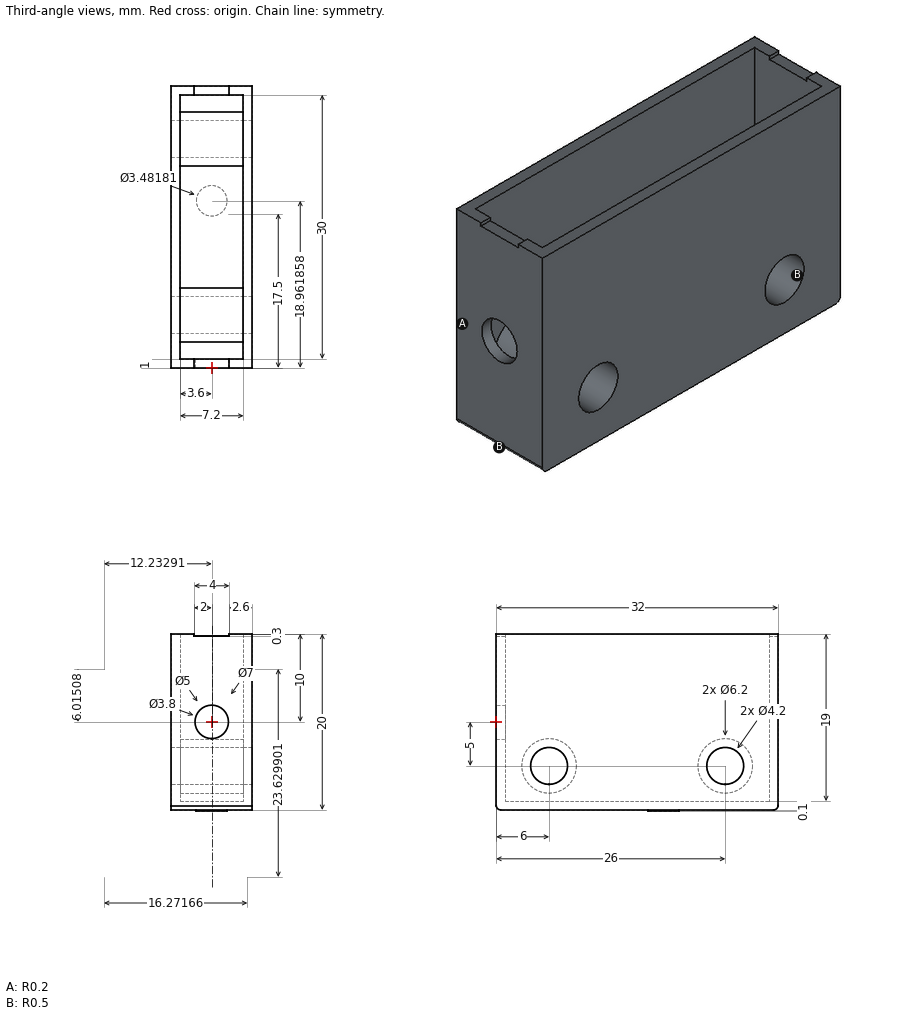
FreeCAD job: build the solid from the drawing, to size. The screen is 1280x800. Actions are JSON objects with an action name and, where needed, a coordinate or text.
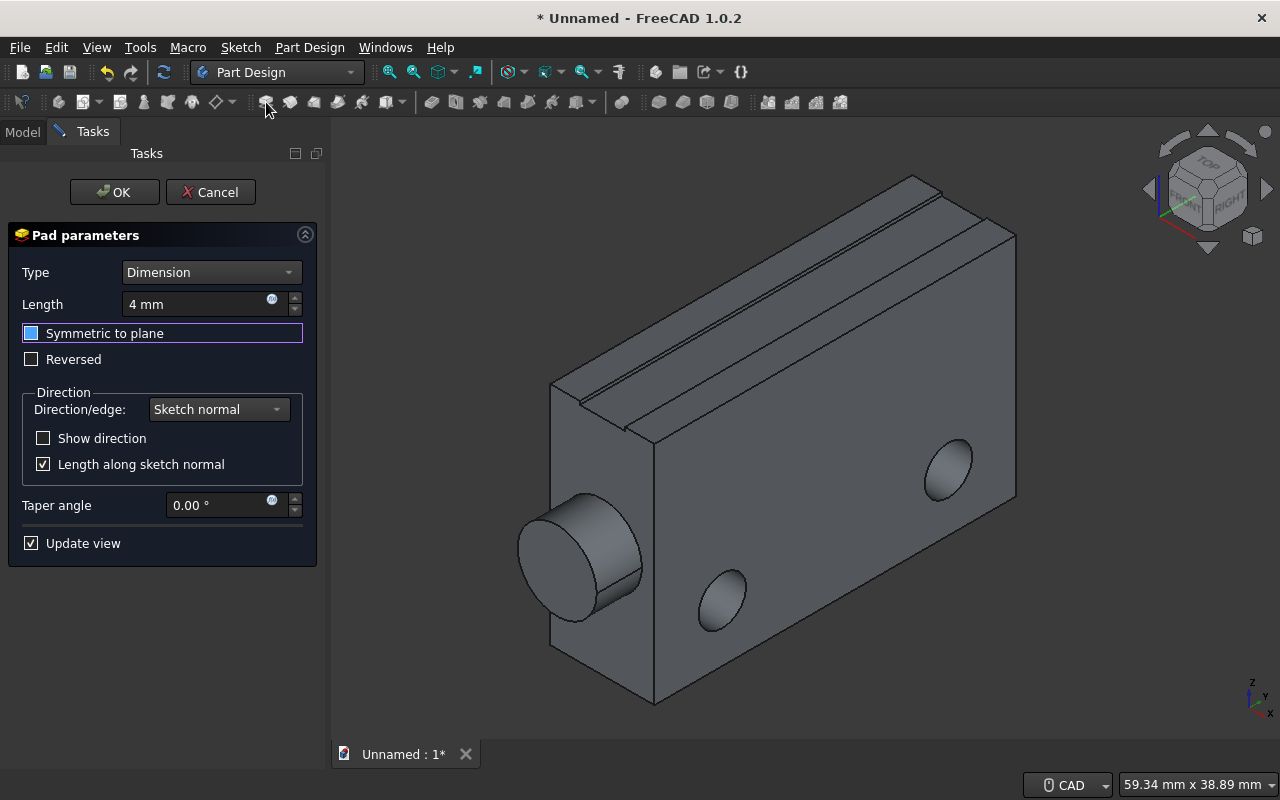
{"action": "left_click", "coordinate": [115, 192]}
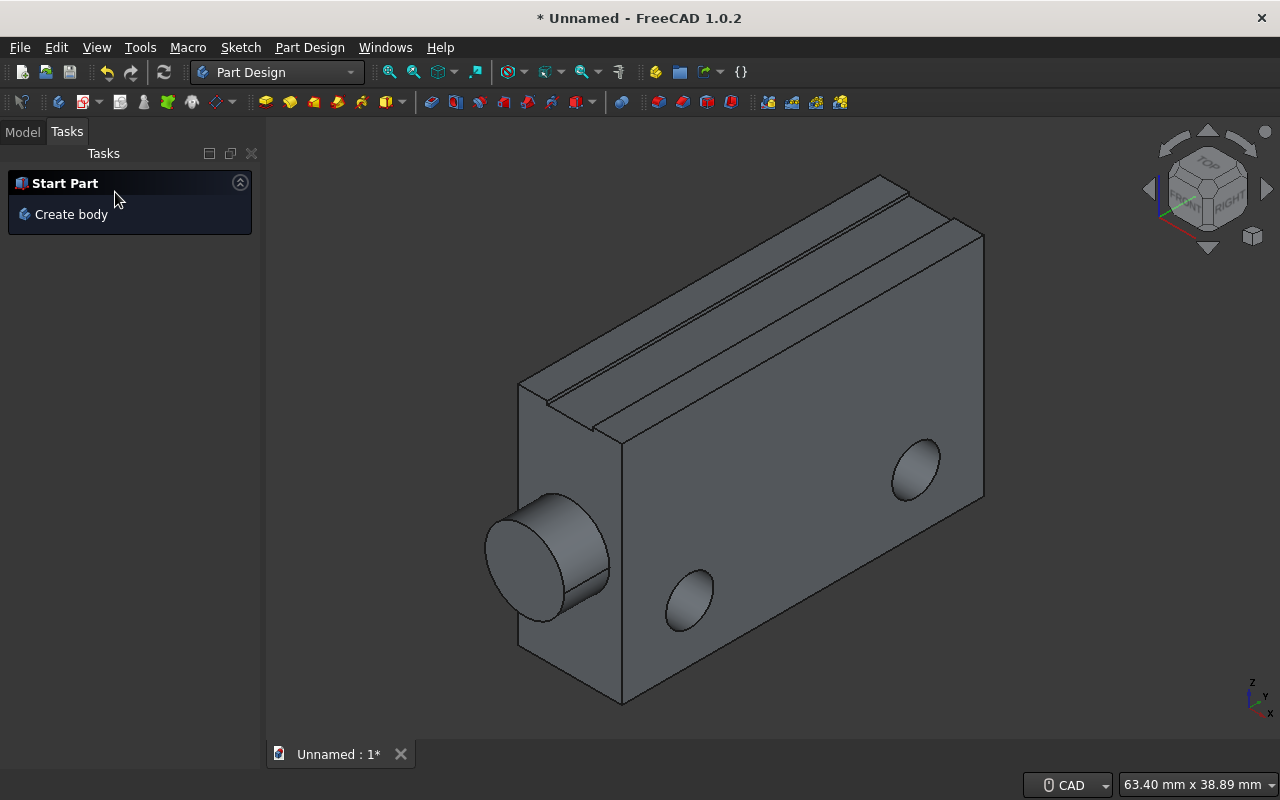
{"action": "left_click", "coordinate": [525, 570]}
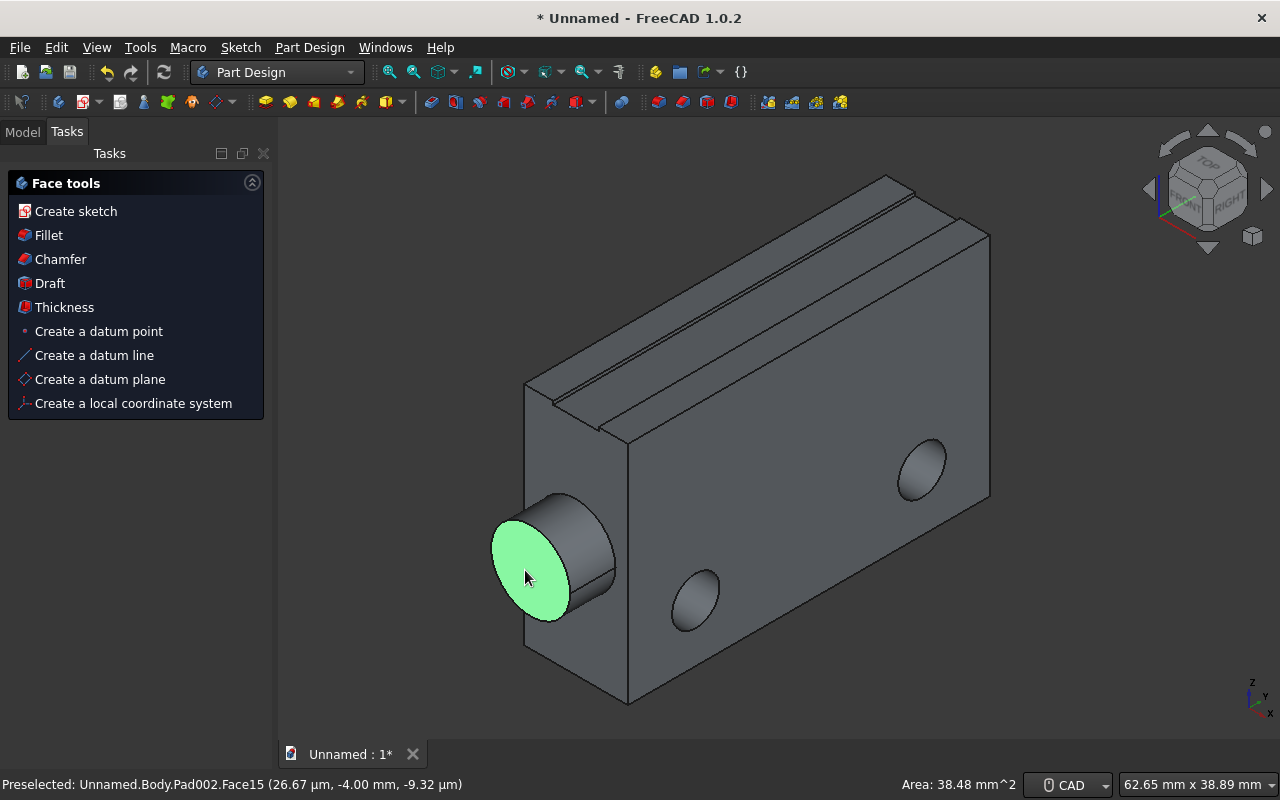
{"action": "left_click", "coordinate": [84, 102]}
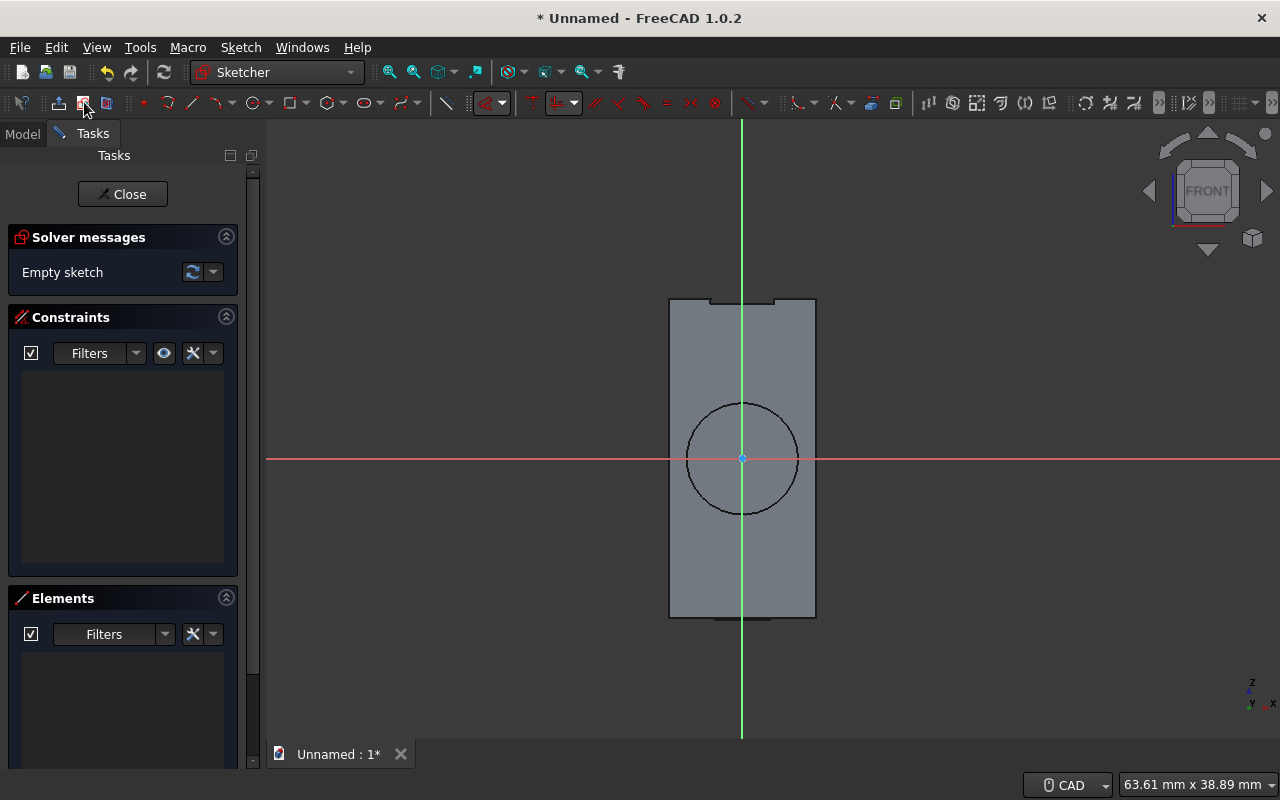
{"action": "scroll", "coordinate": [752, 466], "scroll_direction": "up", "scroll_amount": 8}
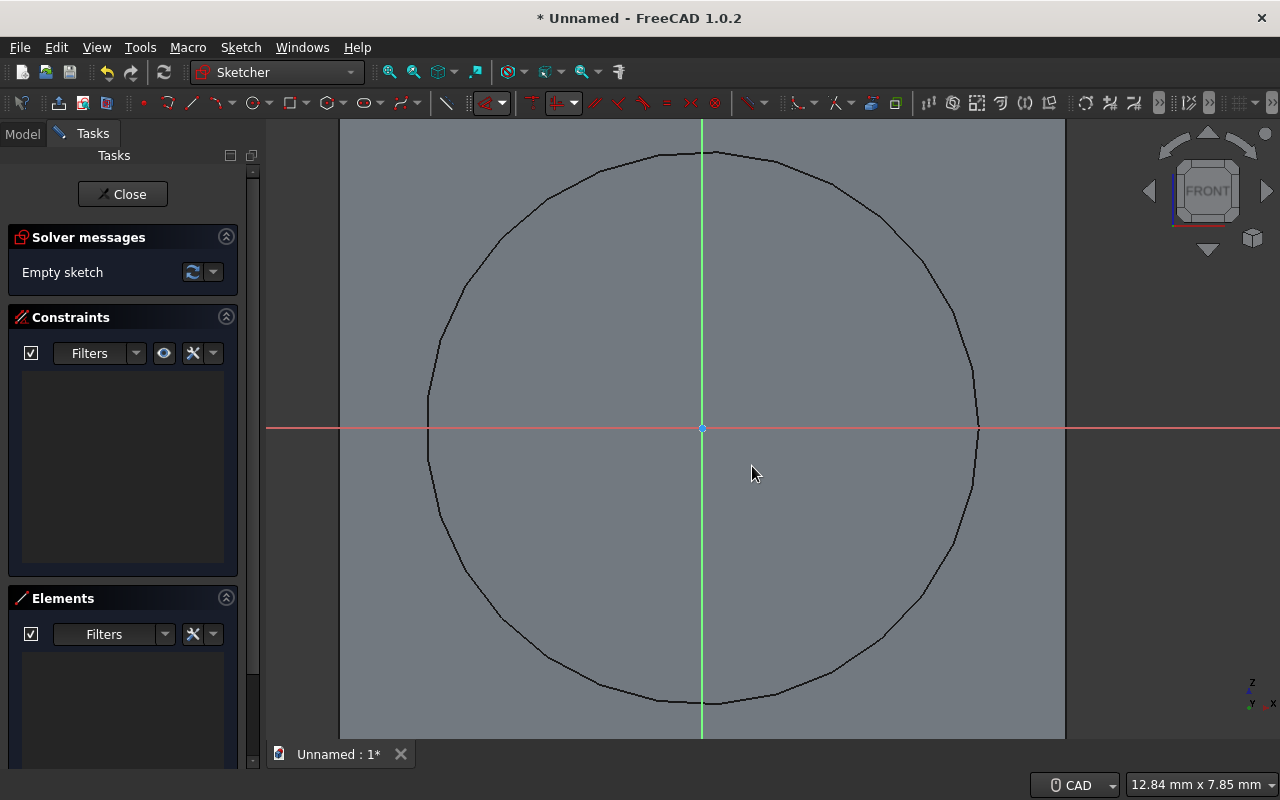
{"action": "left_click", "coordinate": [254, 104]}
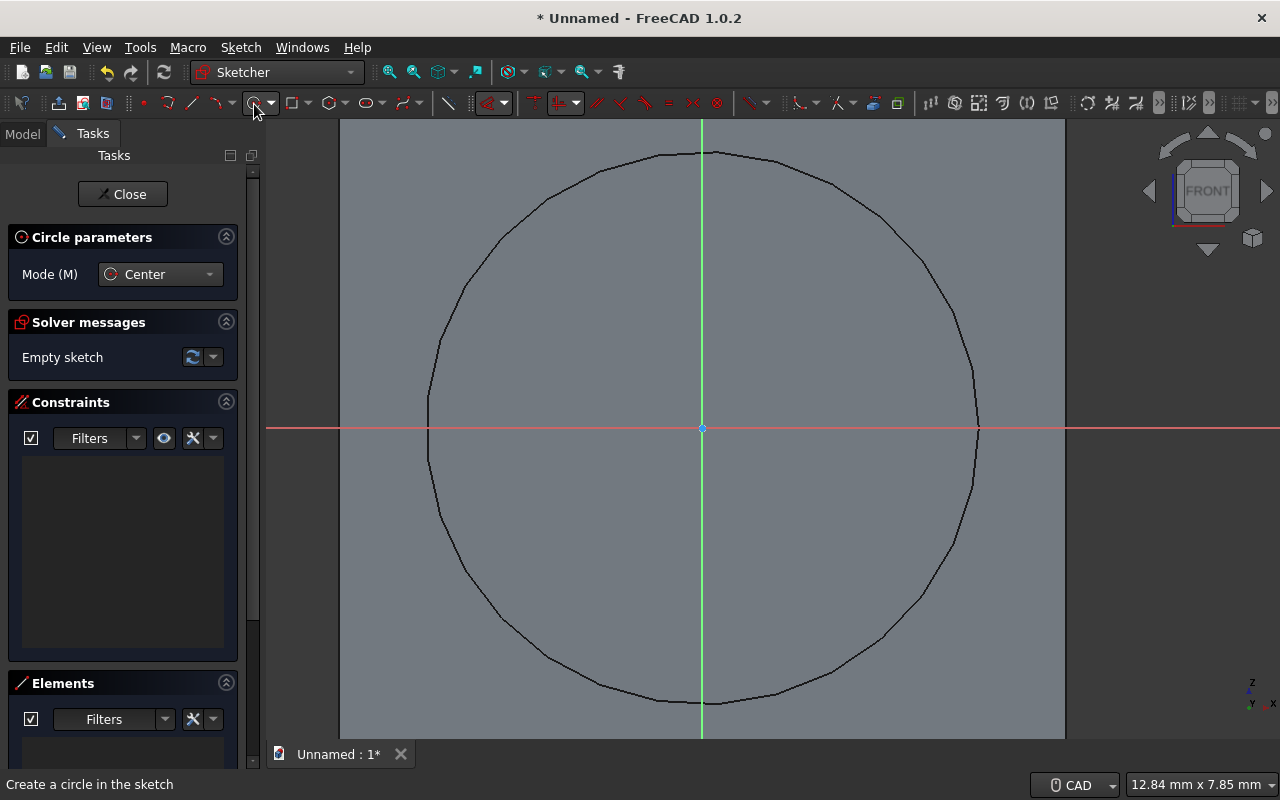
{"action": "left_click", "coordinate": [702, 428]}
{"action": "mouse_move", "coordinate": [842, 289]}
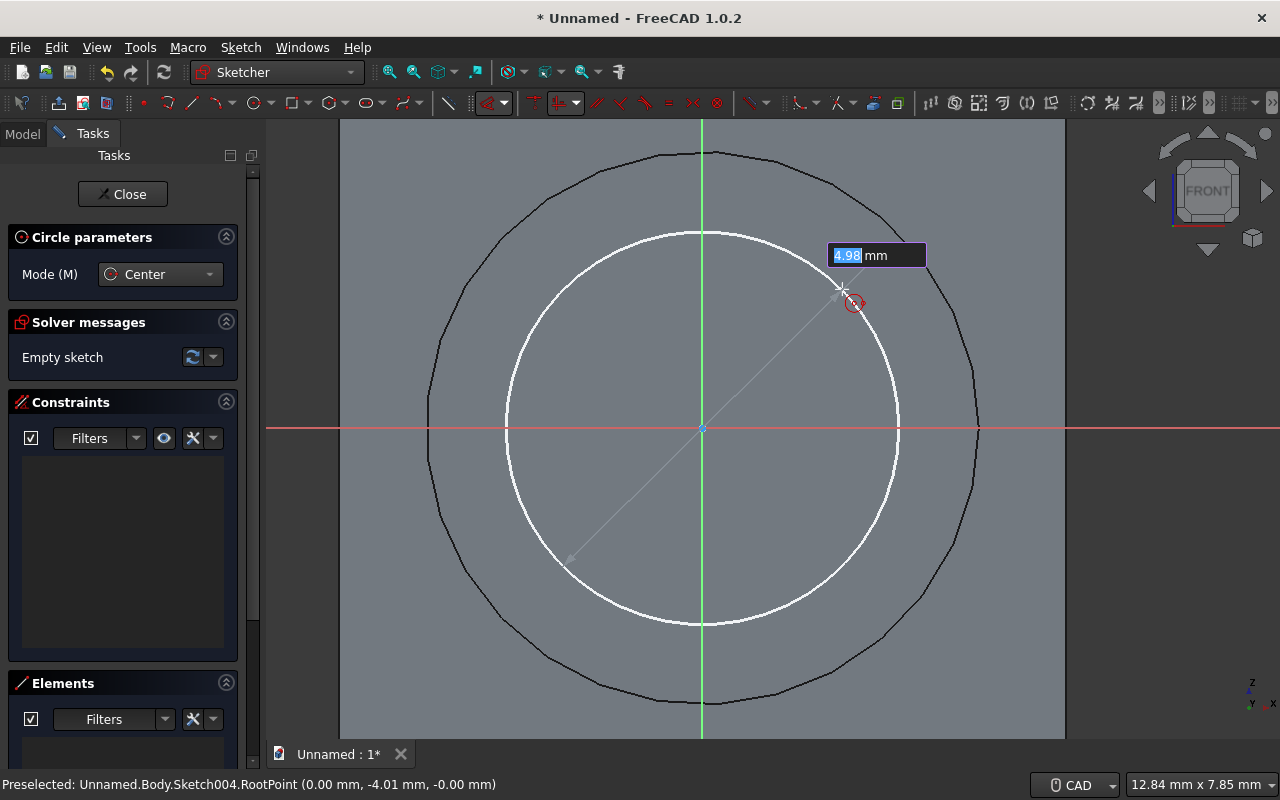
{"action": "type", "text": "5"}
{"action": "key", "text": "Return"}
{"action": "key", "text": "Escape"}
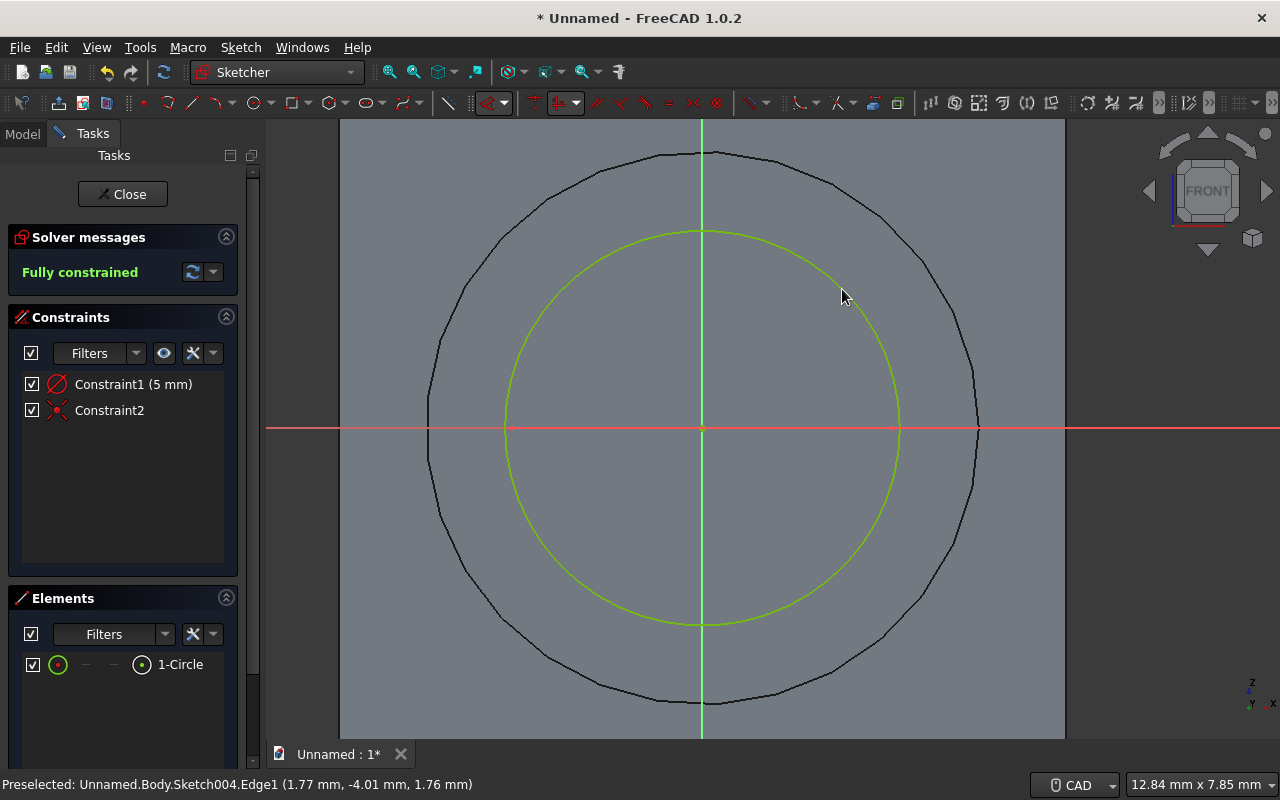
{"action": "left_click", "coordinate": [123, 194]}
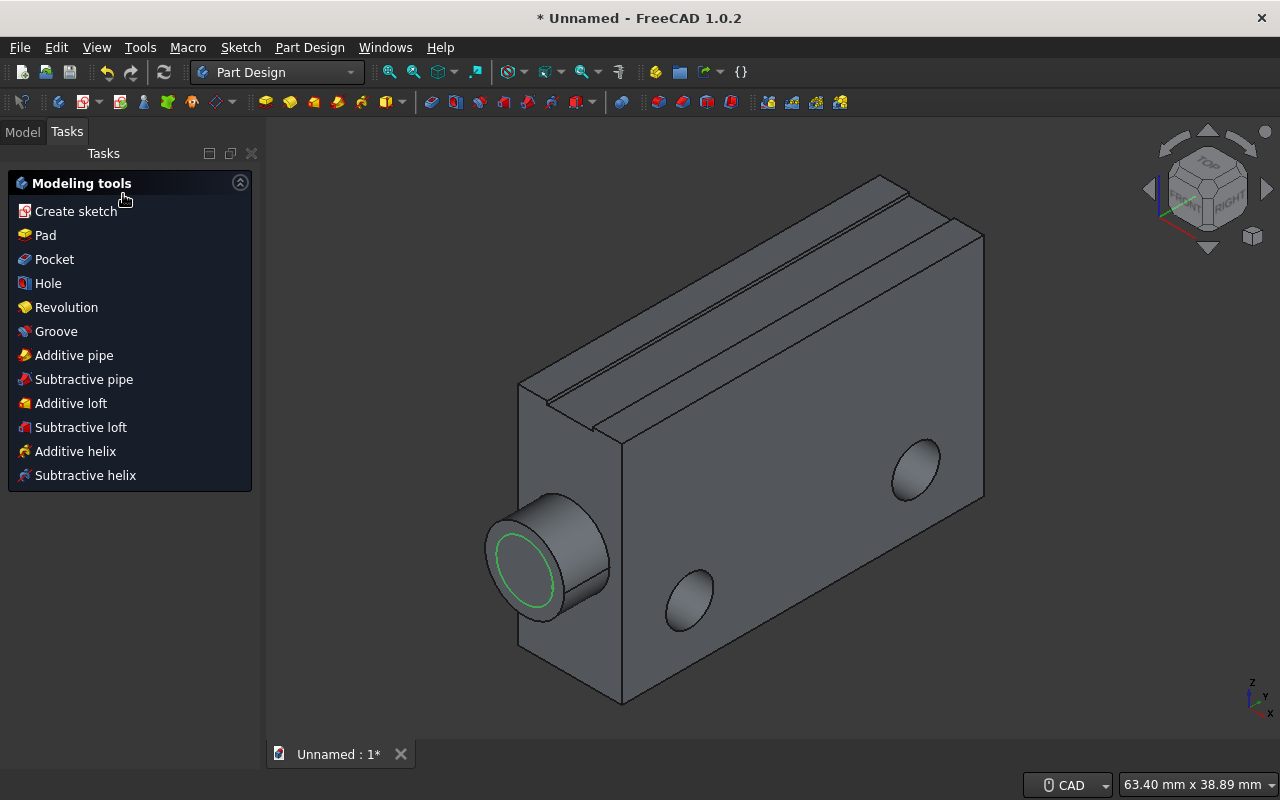
{"action": "left_click", "coordinate": [266, 102]}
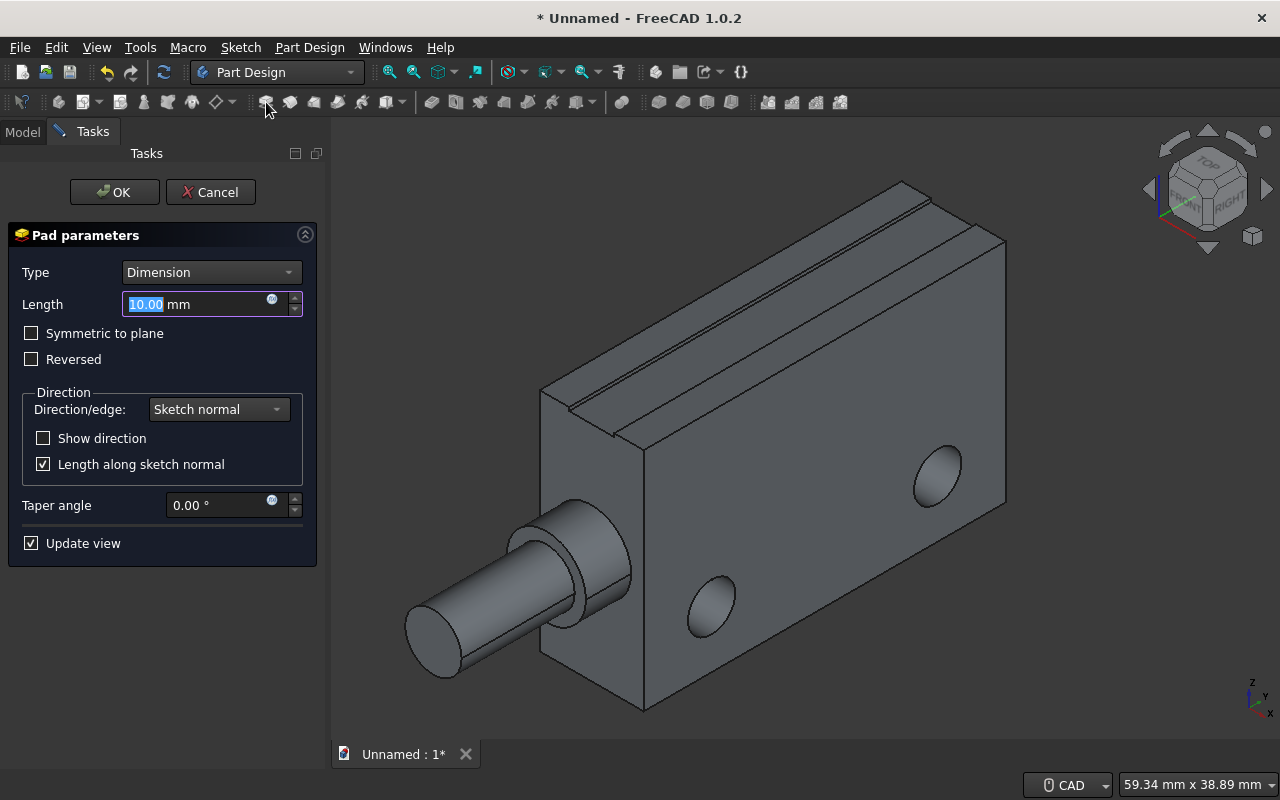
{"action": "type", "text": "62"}
{"action": "key", "text": "Tab"}